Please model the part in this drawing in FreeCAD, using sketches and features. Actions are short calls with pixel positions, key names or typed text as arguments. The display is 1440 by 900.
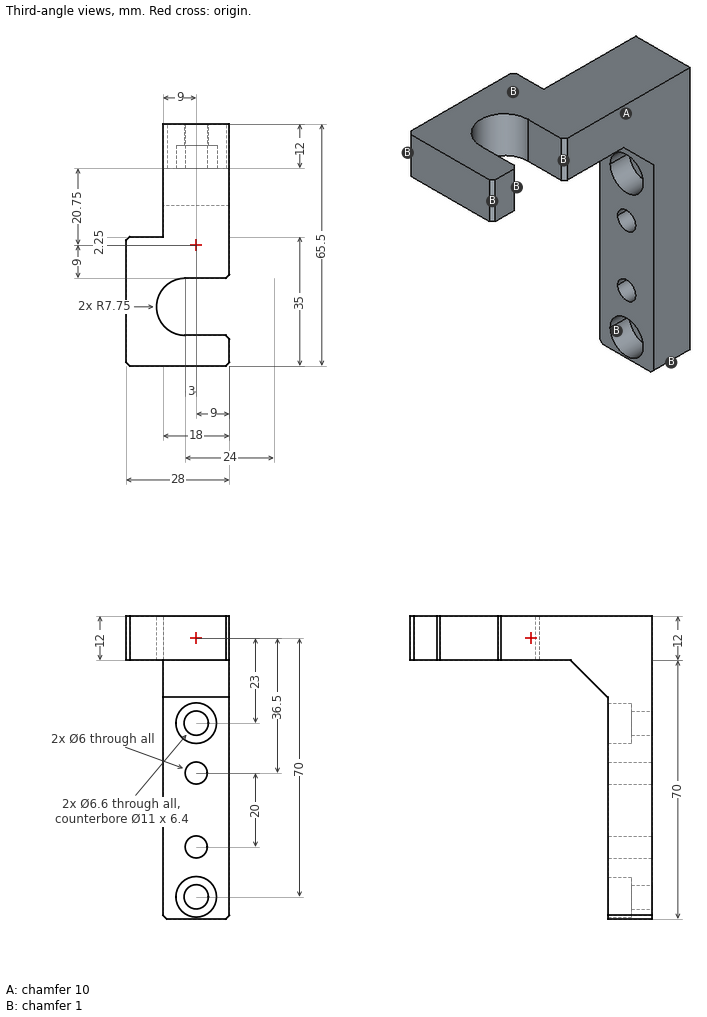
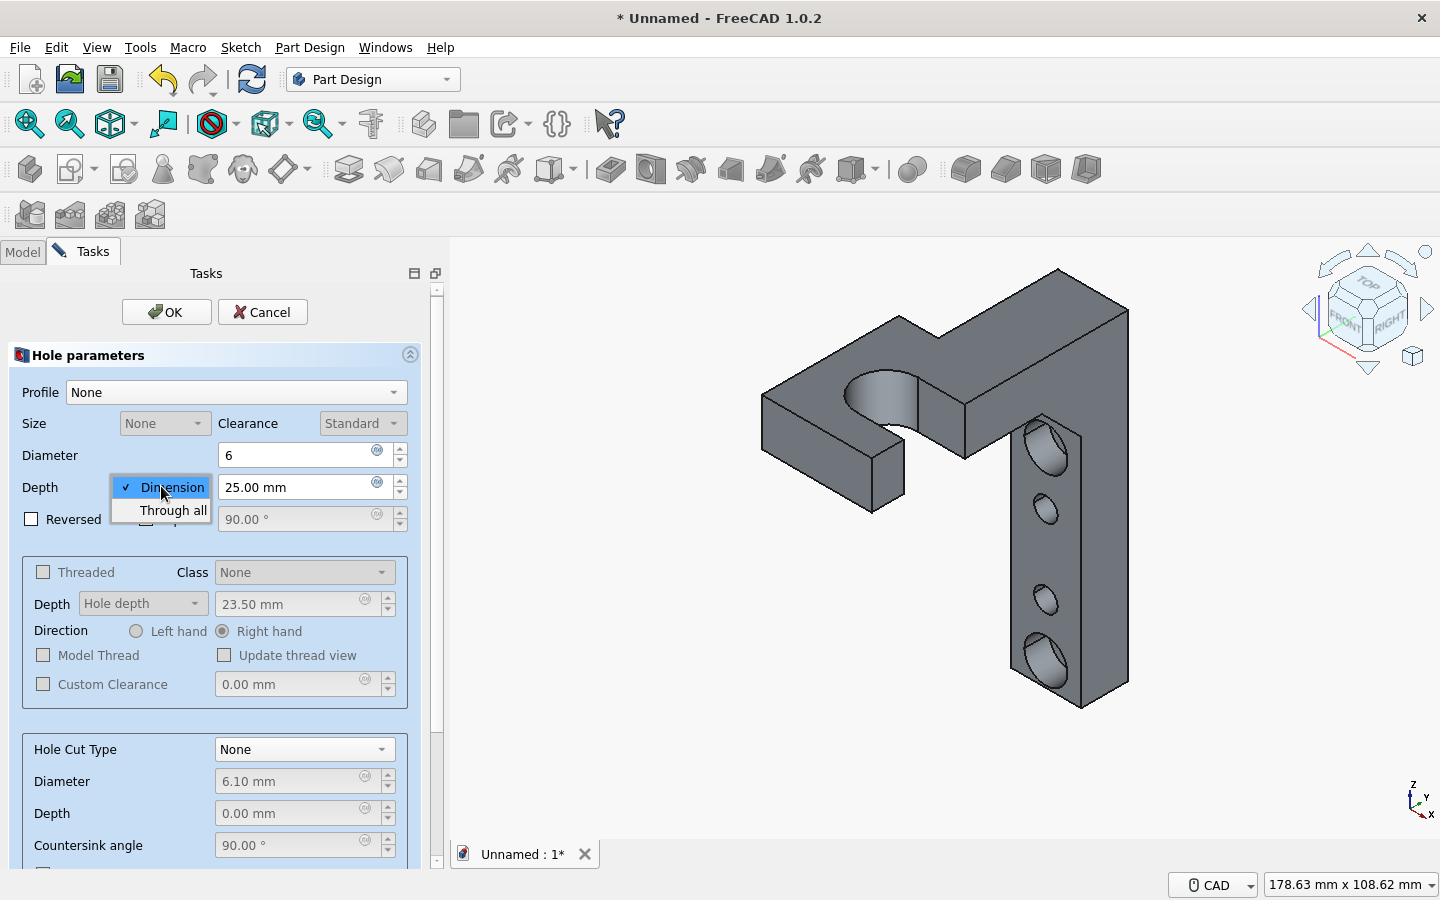
click(160, 510)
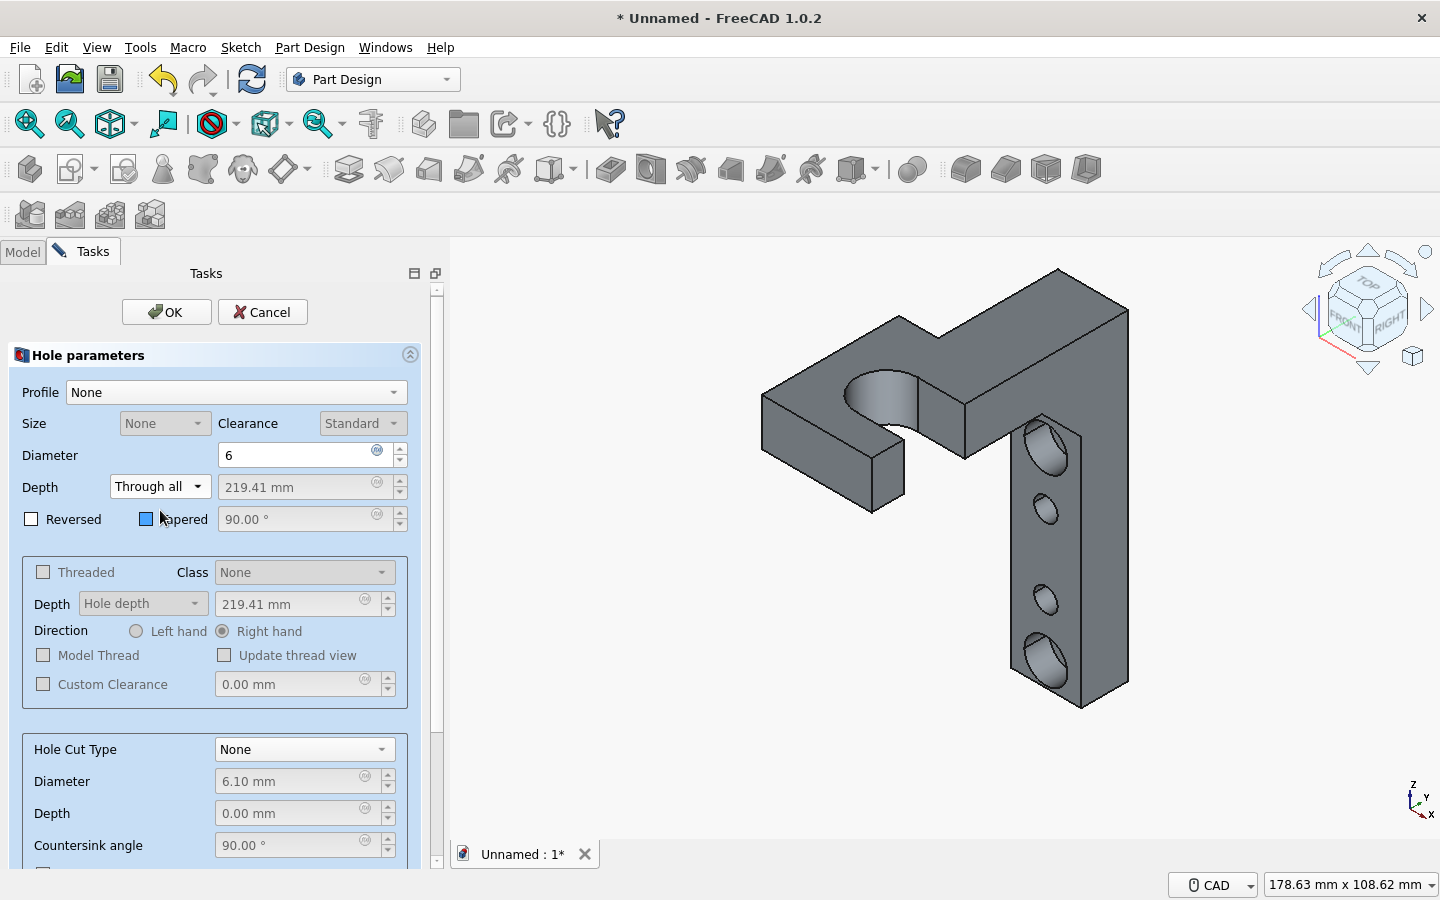
click(167, 312)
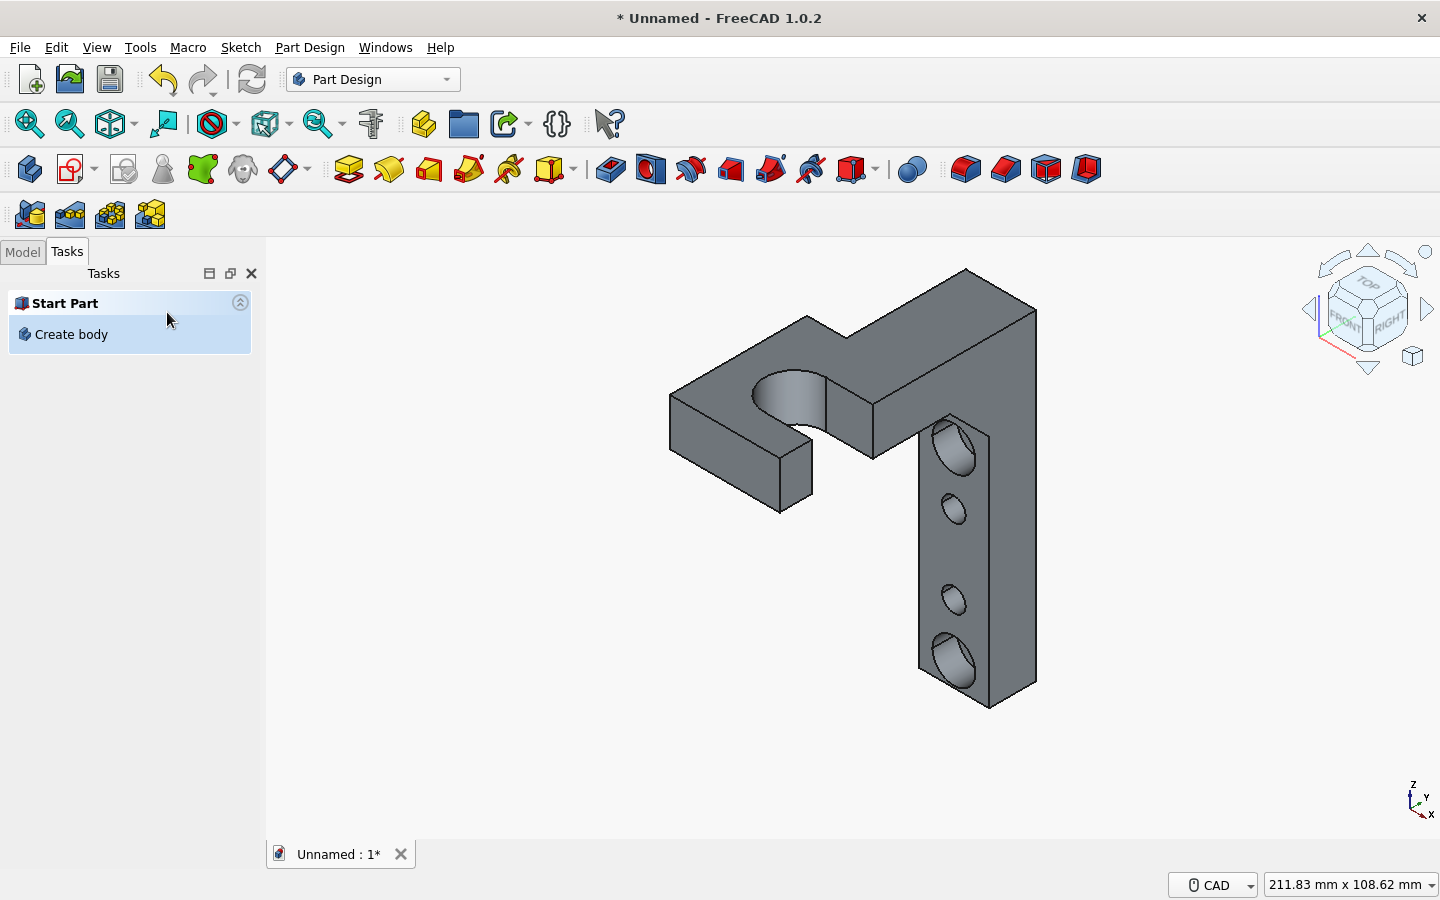
click(873, 431)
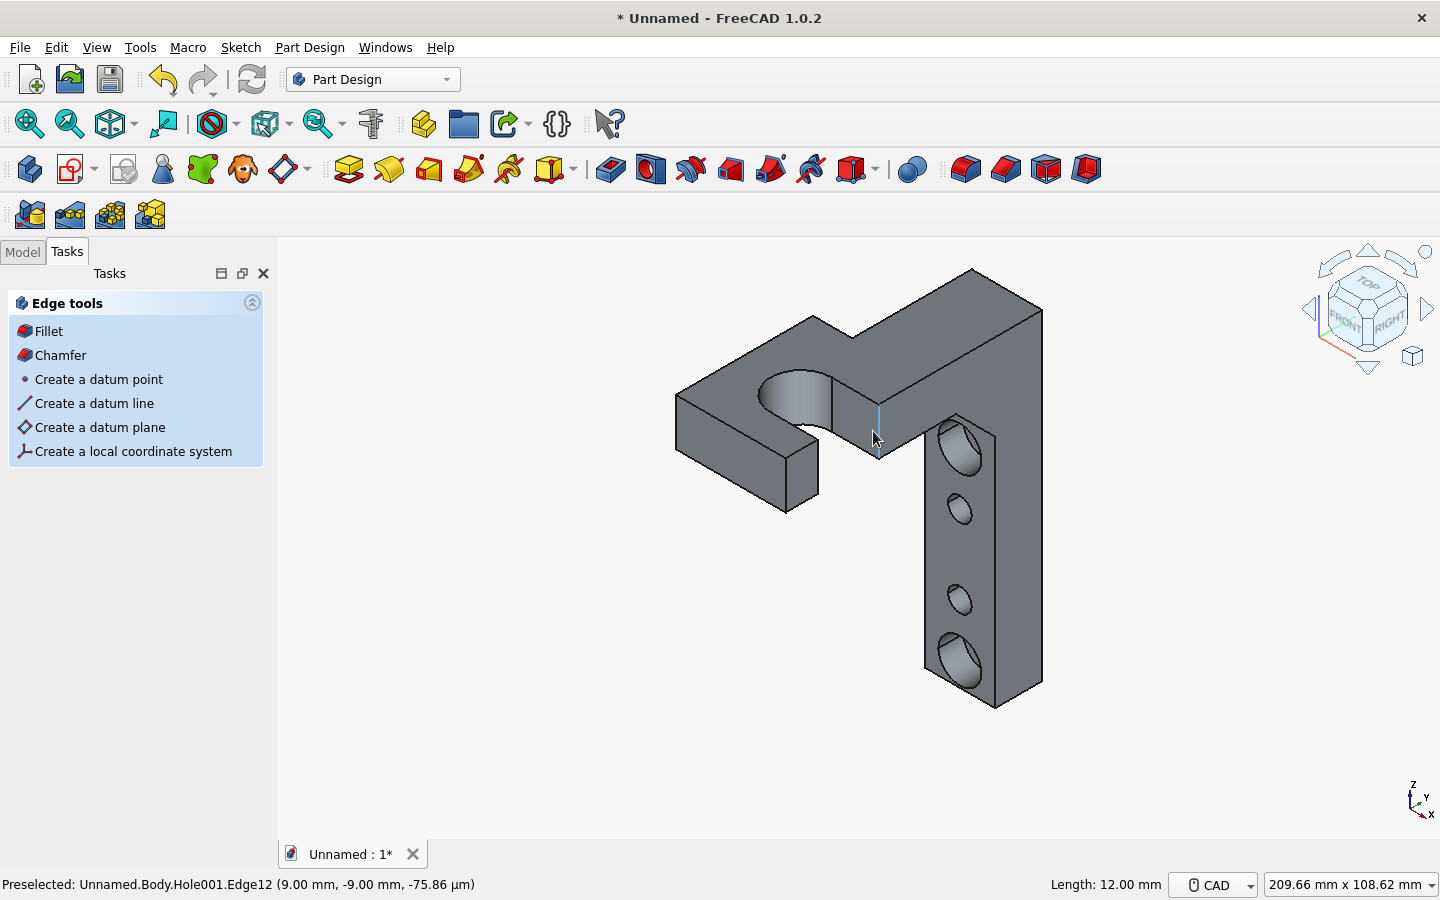
click(786, 484, ctrl)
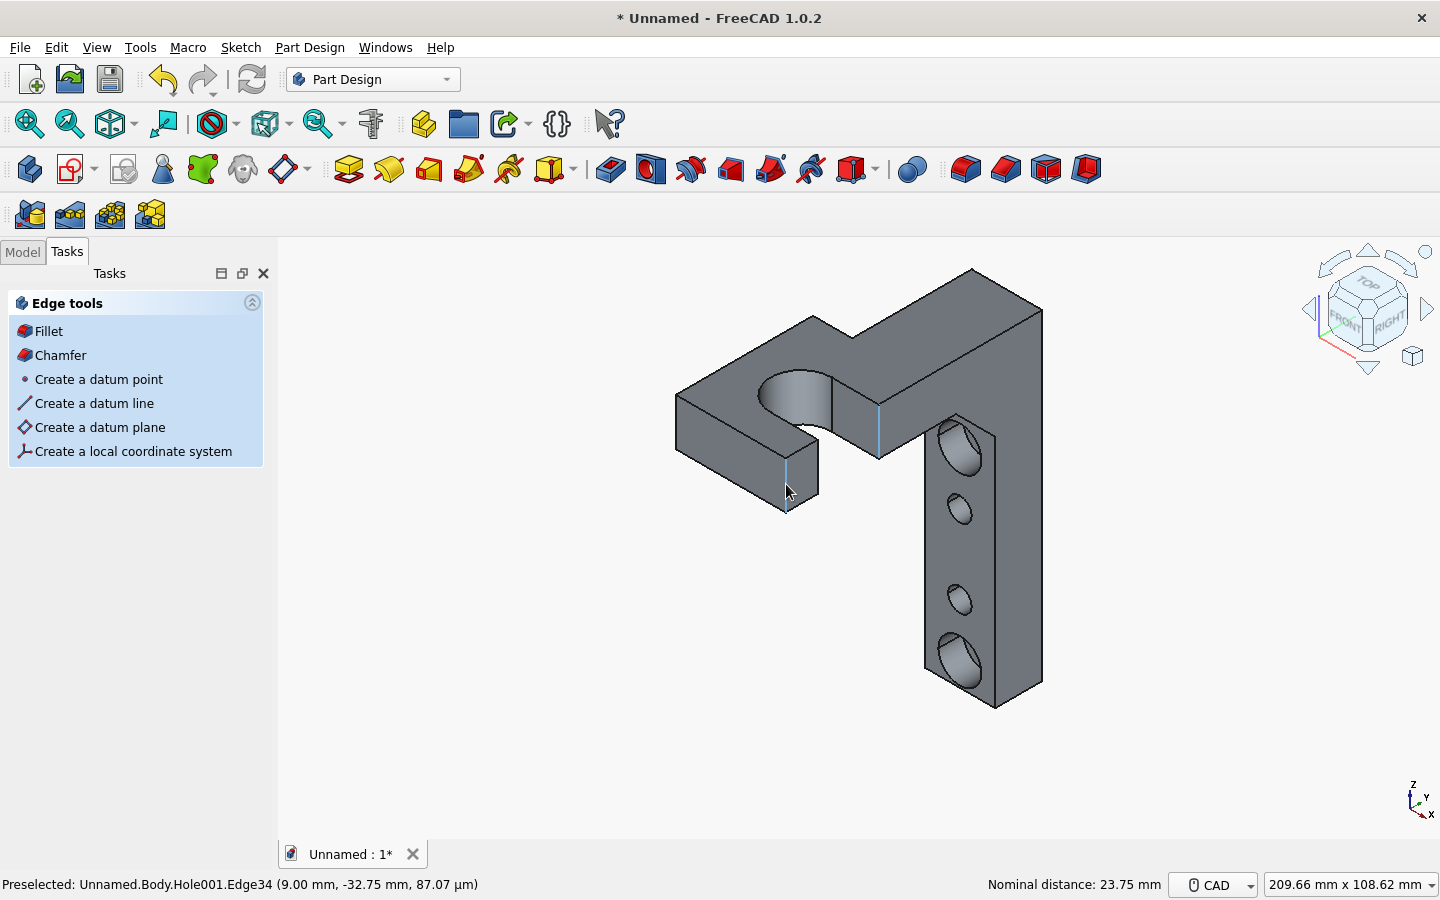
key(2)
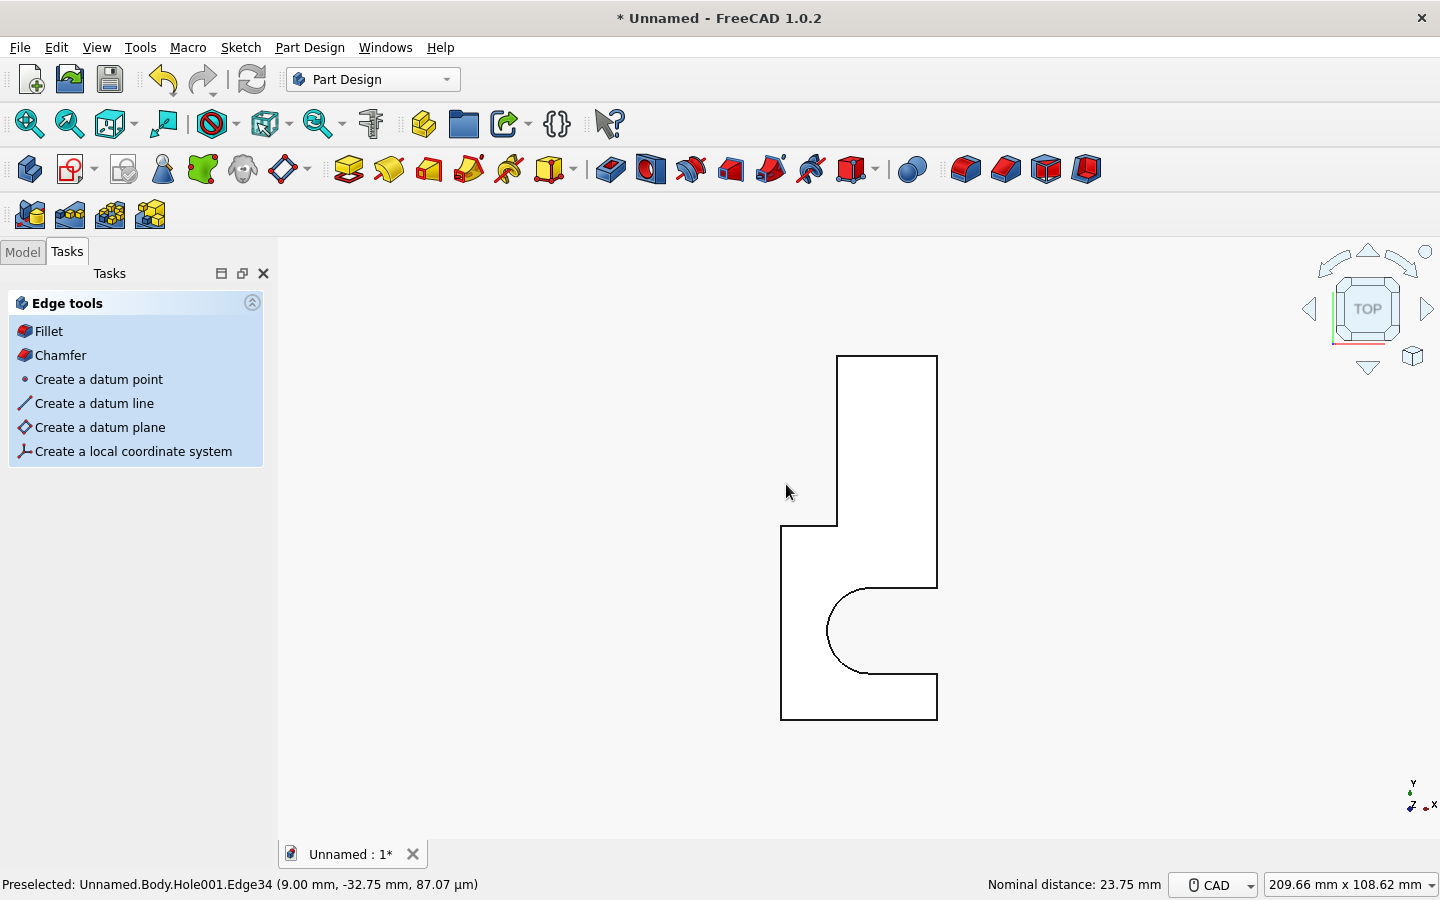
key(0)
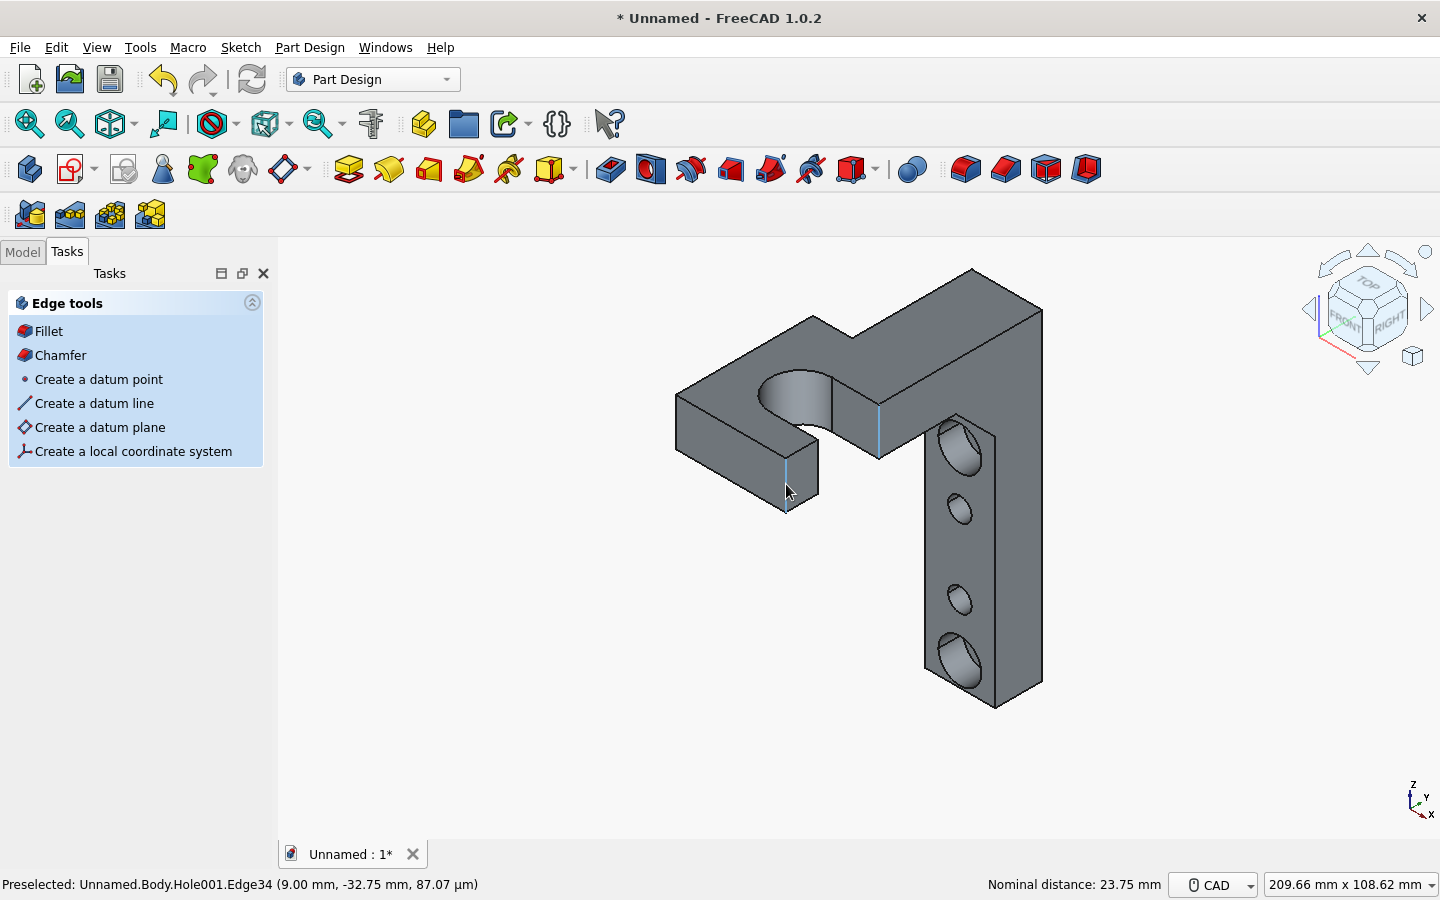
key(1)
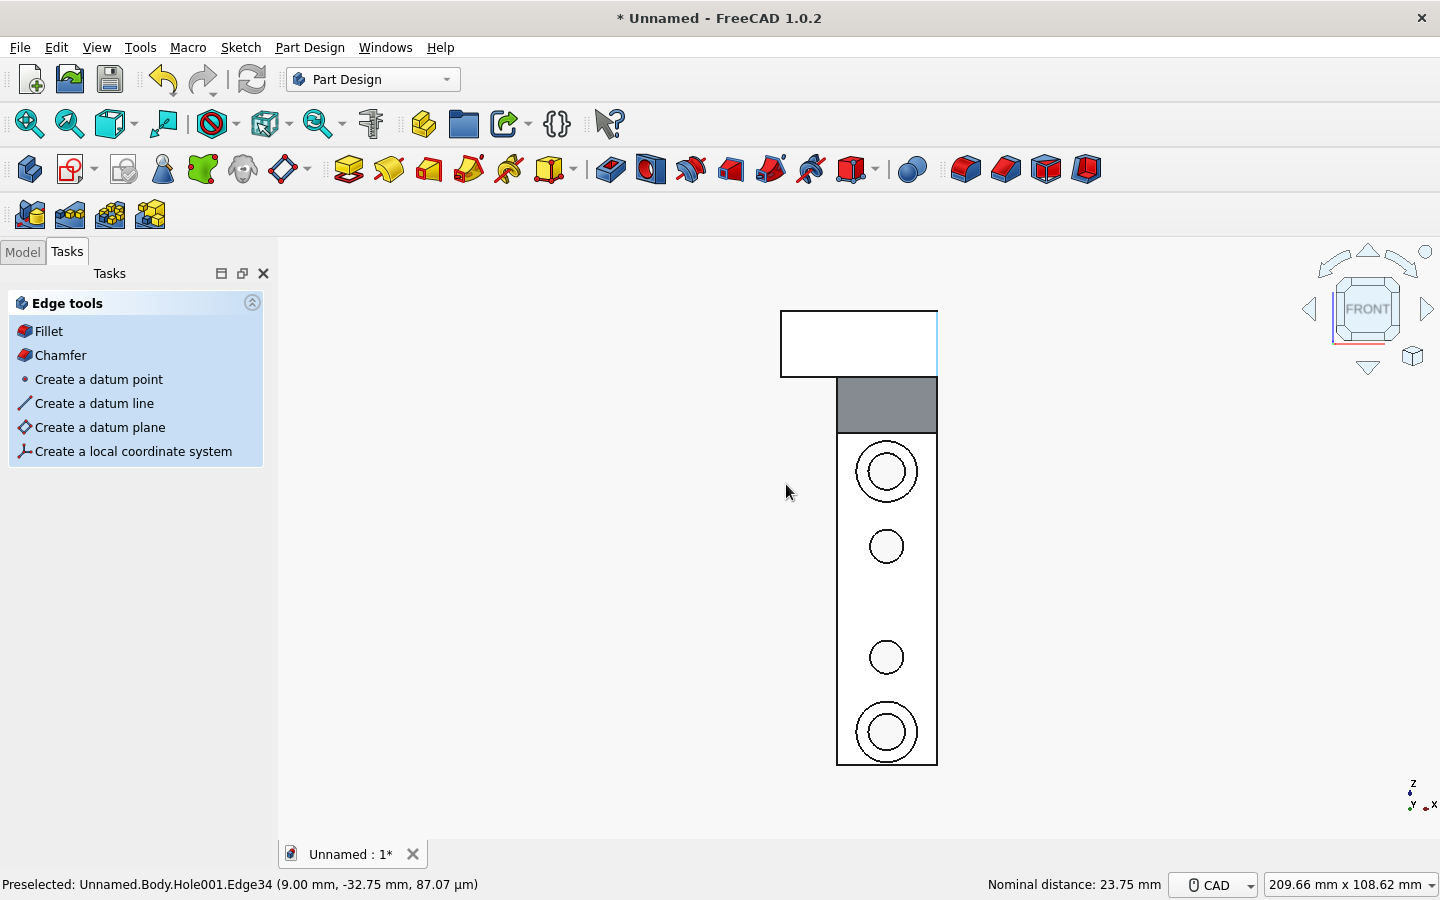
click(781, 343, ctrl)